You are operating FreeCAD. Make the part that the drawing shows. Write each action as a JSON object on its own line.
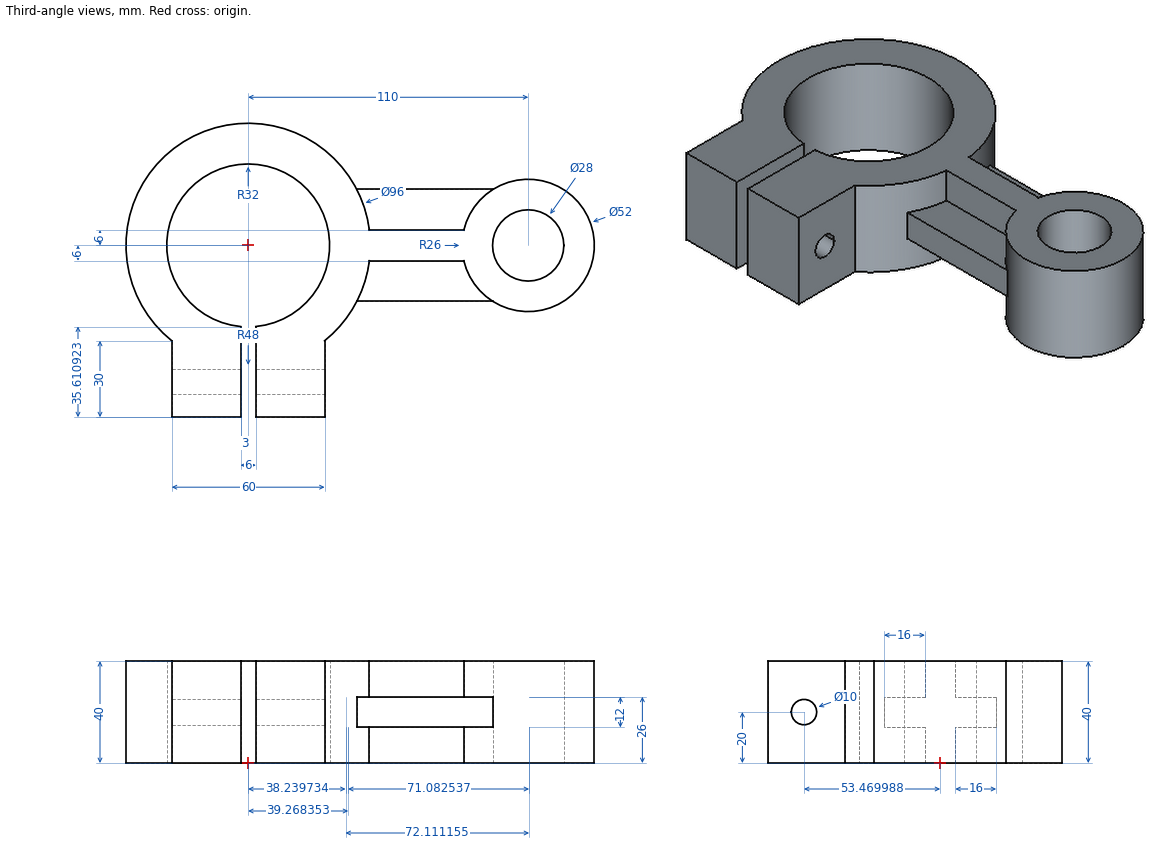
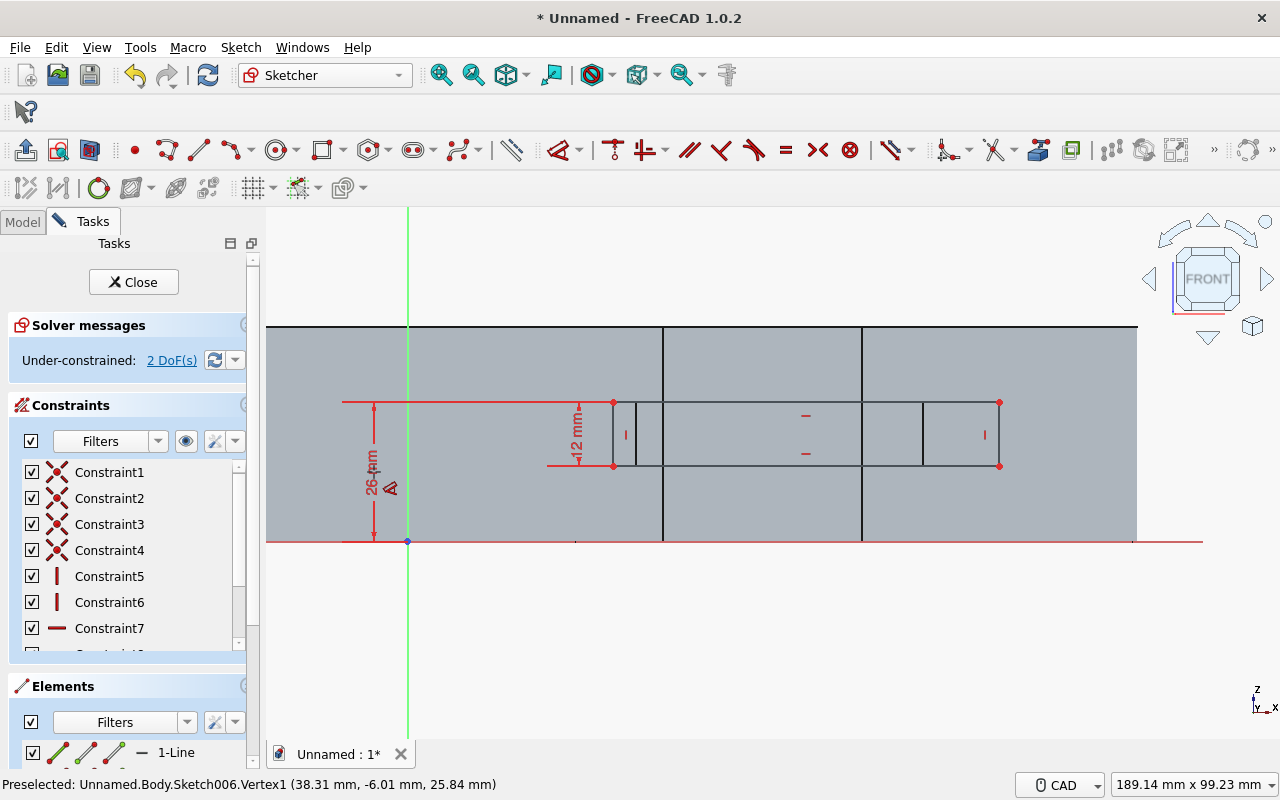
{"action": "left_click", "coordinate": [729, 466]}
{"action": "left_click", "coordinate": [806, 432]}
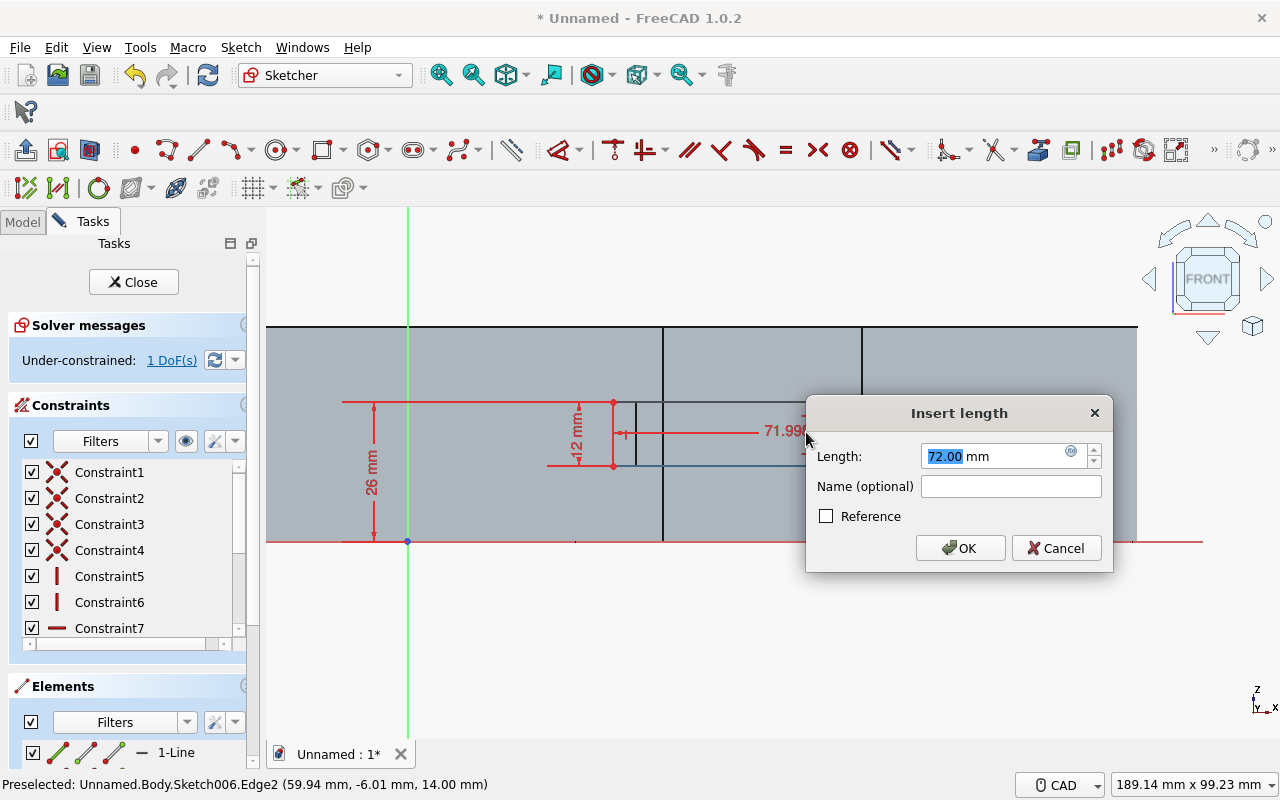
{"action": "type", "text": "72.111155"}
{"action": "key", "text": "Return"}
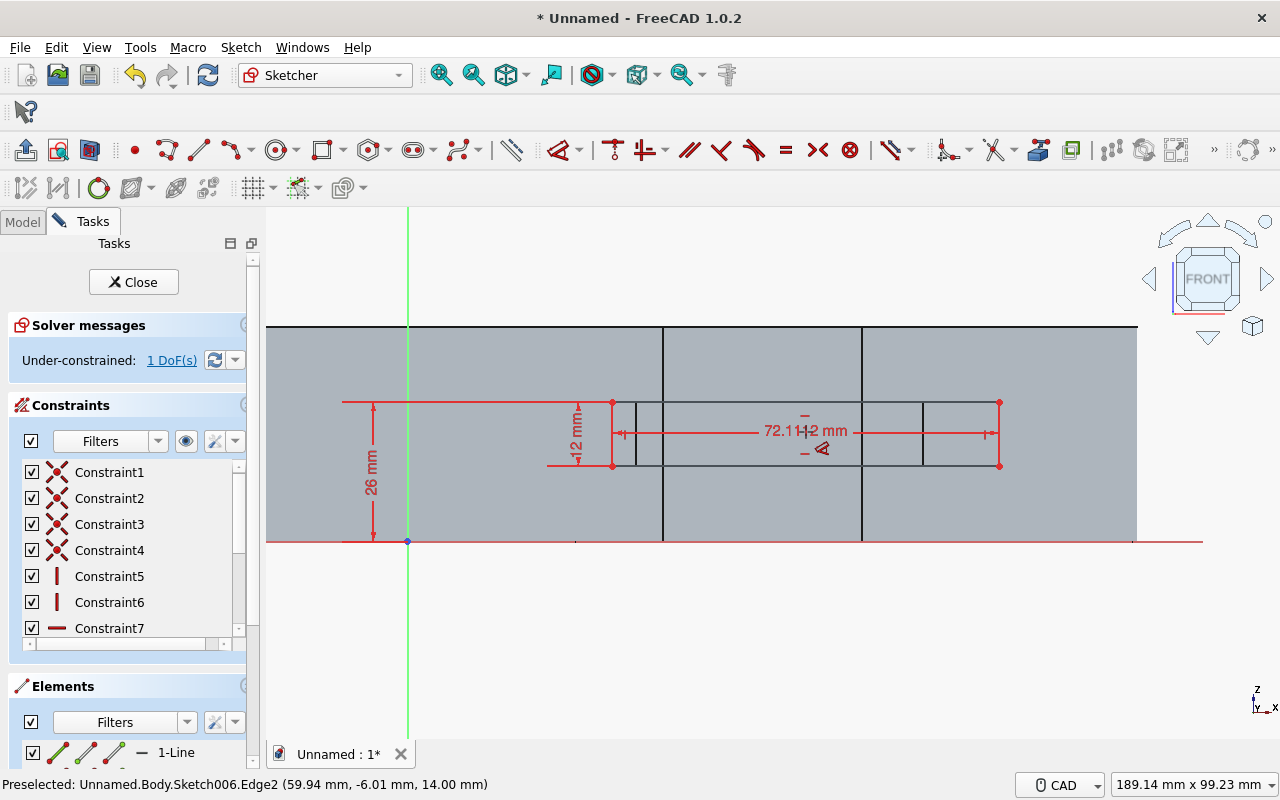
{"action": "left_click", "coordinate": [612, 402]}
{"action": "left_click", "coordinate": [510, 576]}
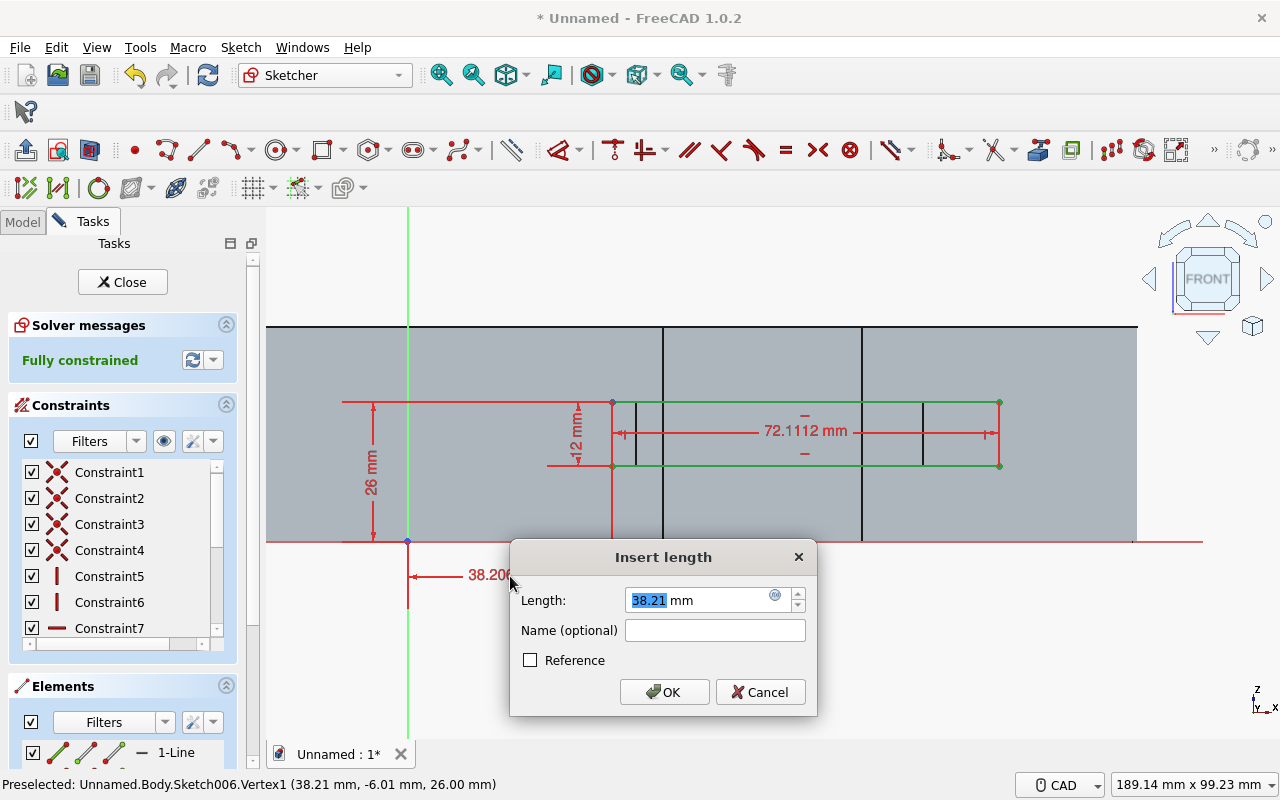
{"action": "type", "text": "38.239734"}
{"action": "key", "text": "Return"}
{"action": "key", "text": "Escape"}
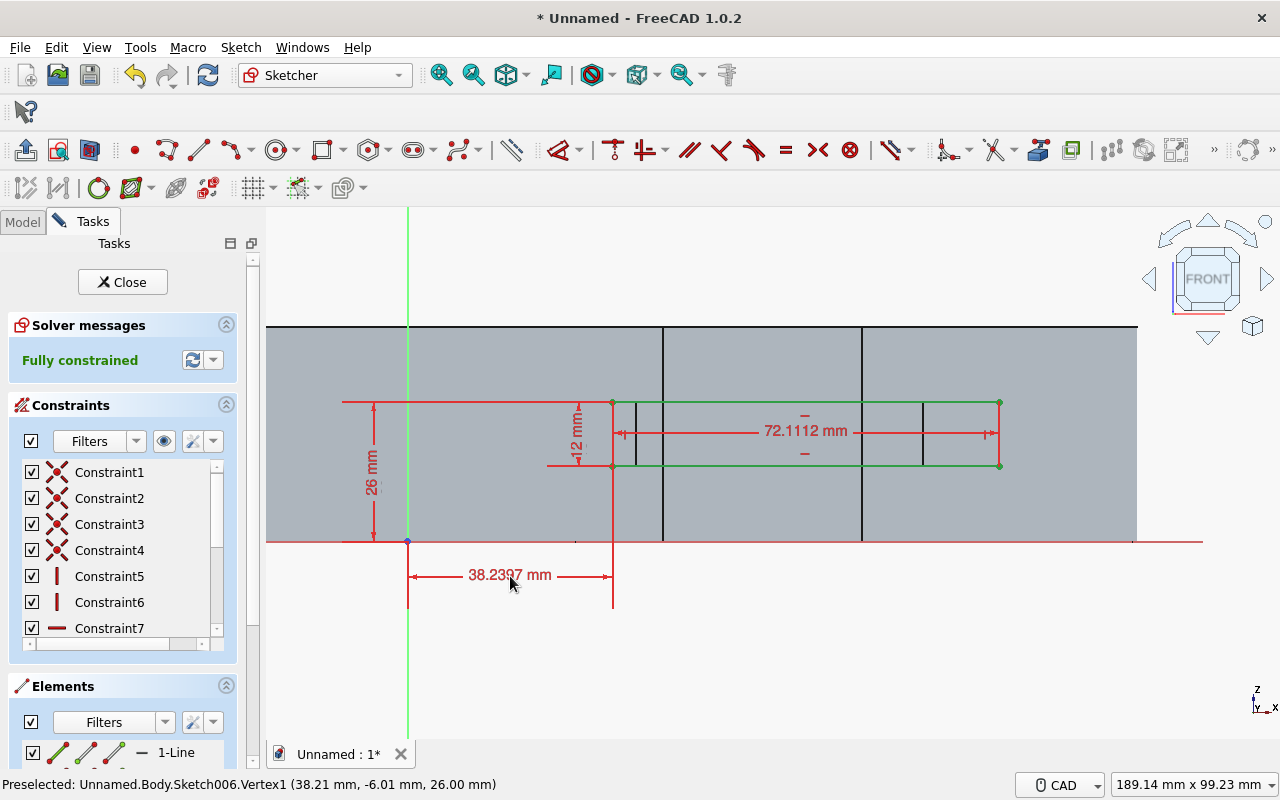
{"action": "left_click", "coordinate": [123, 282]}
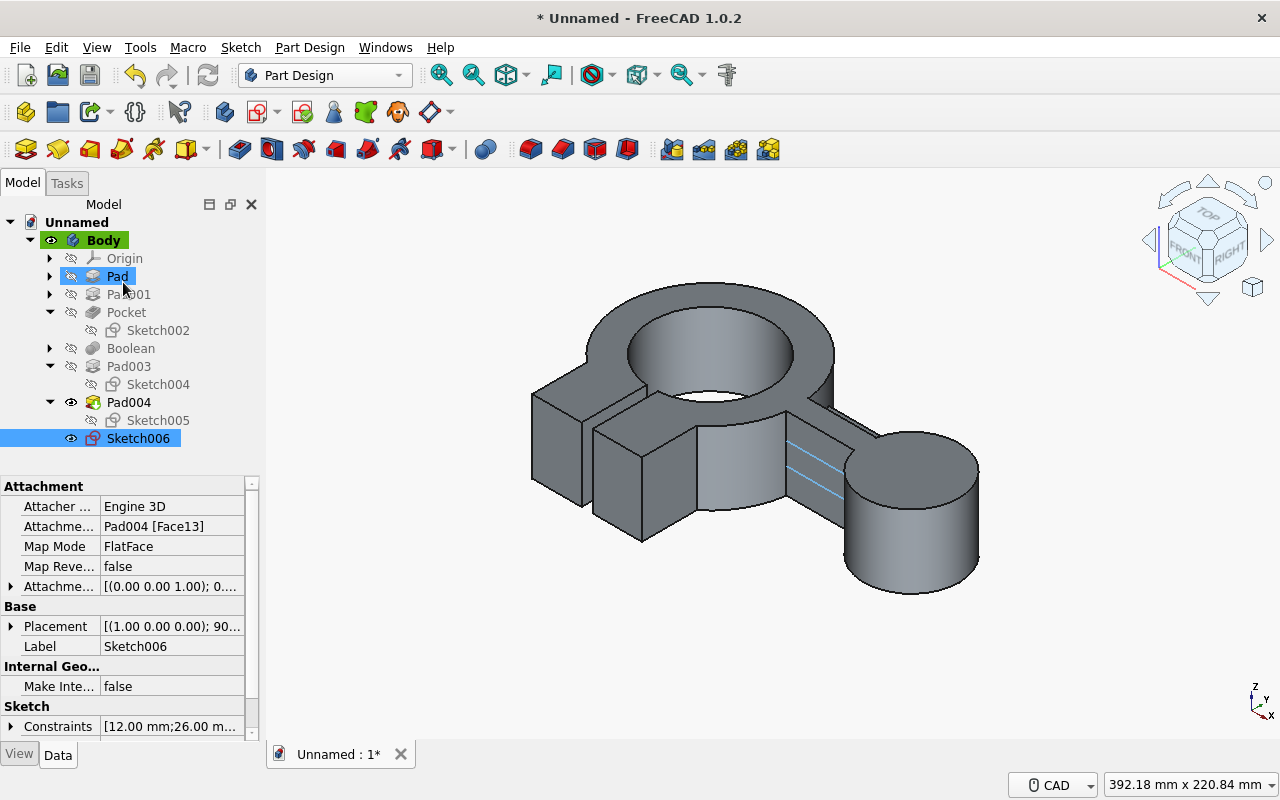
{"action": "left_click", "coordinate": [26, 150]}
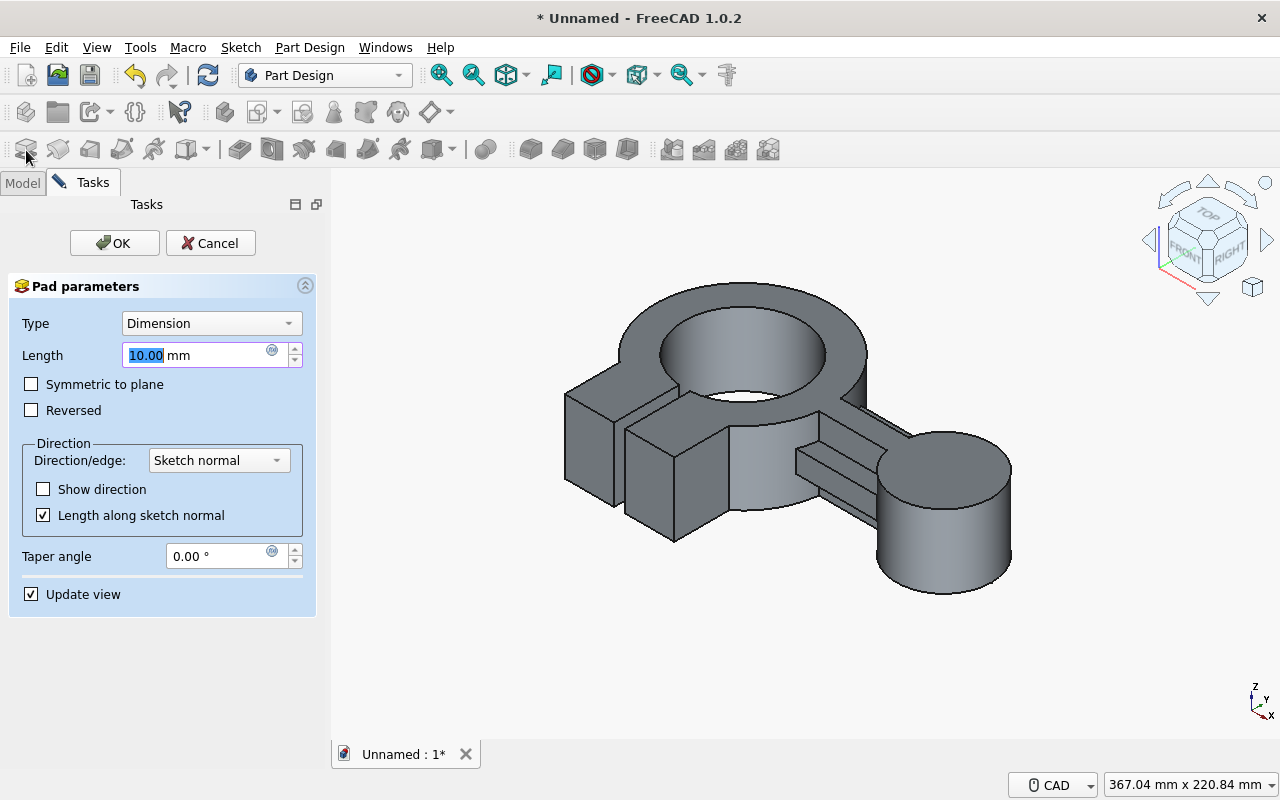
{"action": "type", "text": "16"}
{"action": "key", "text": "Tab"}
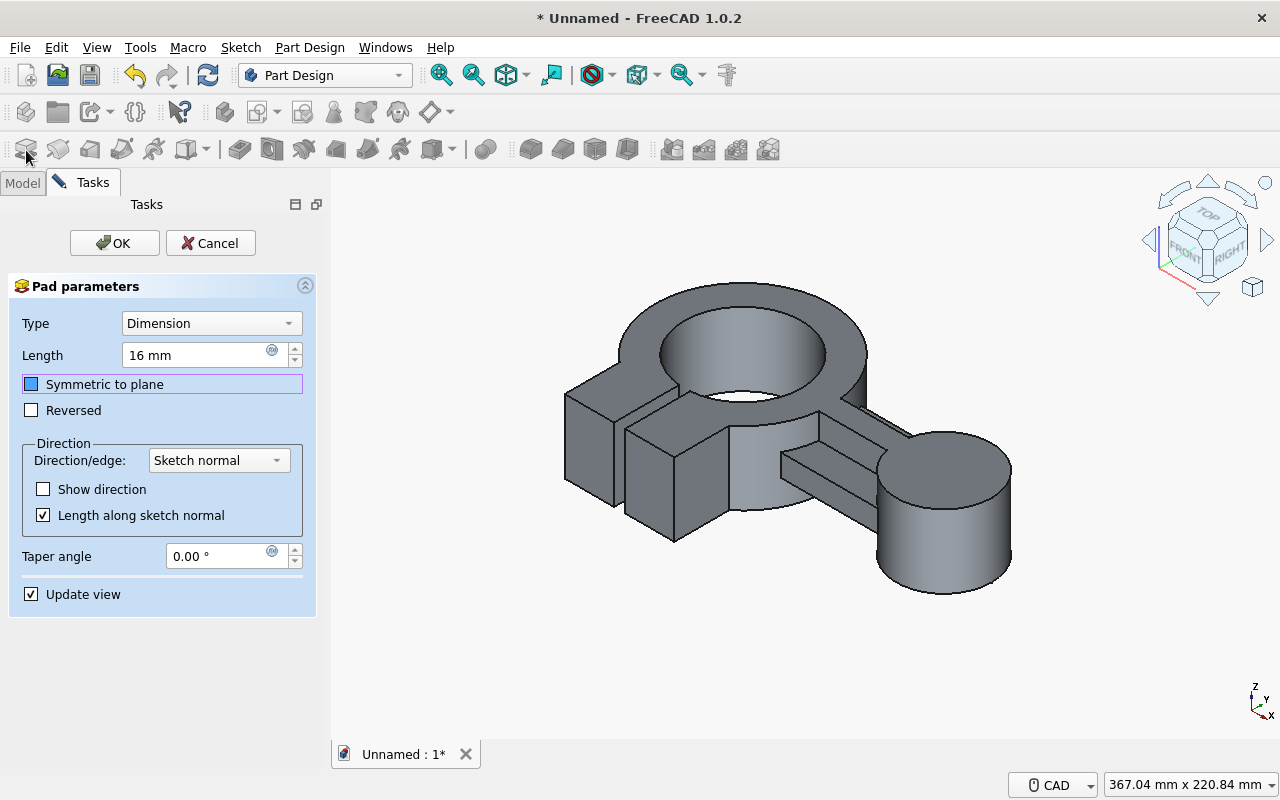
{"action": "left_click", "coordinate": [115, 243]}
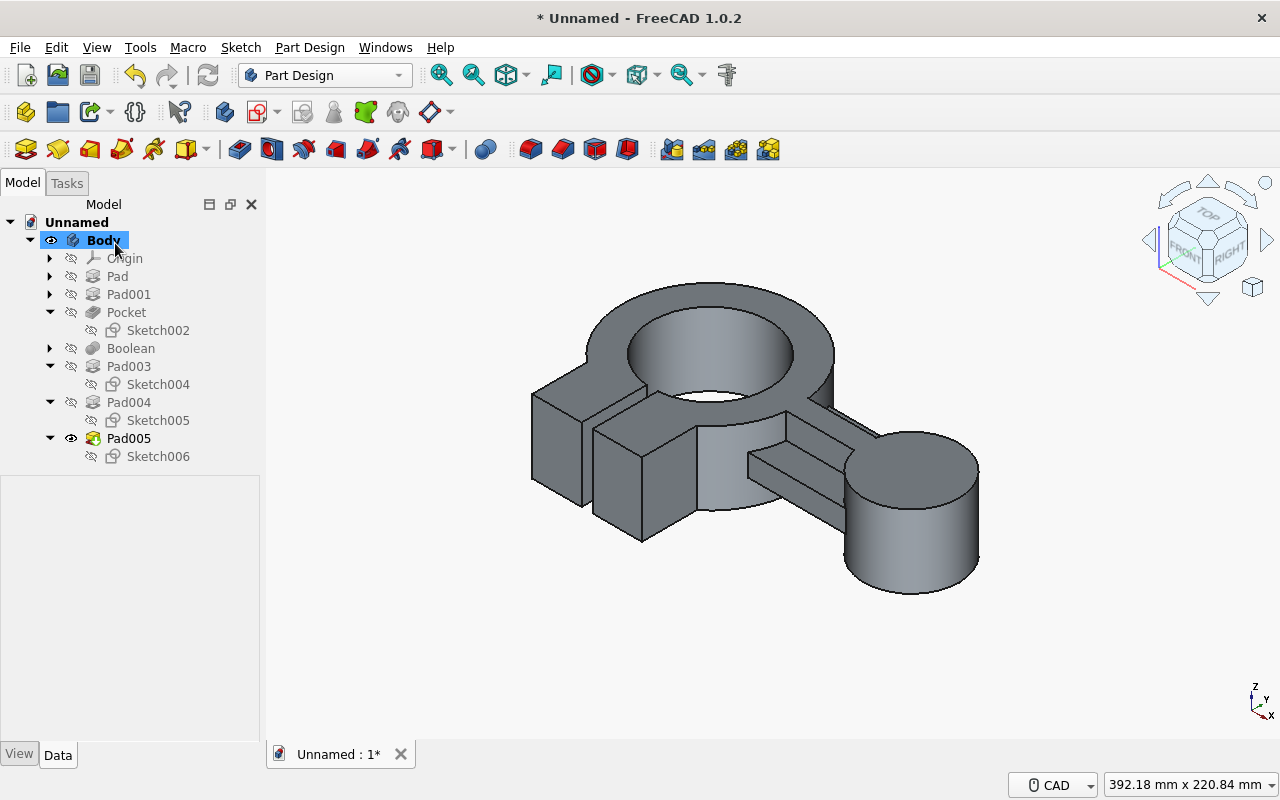
{"action": "left_click", "coordinate": [665, 417]}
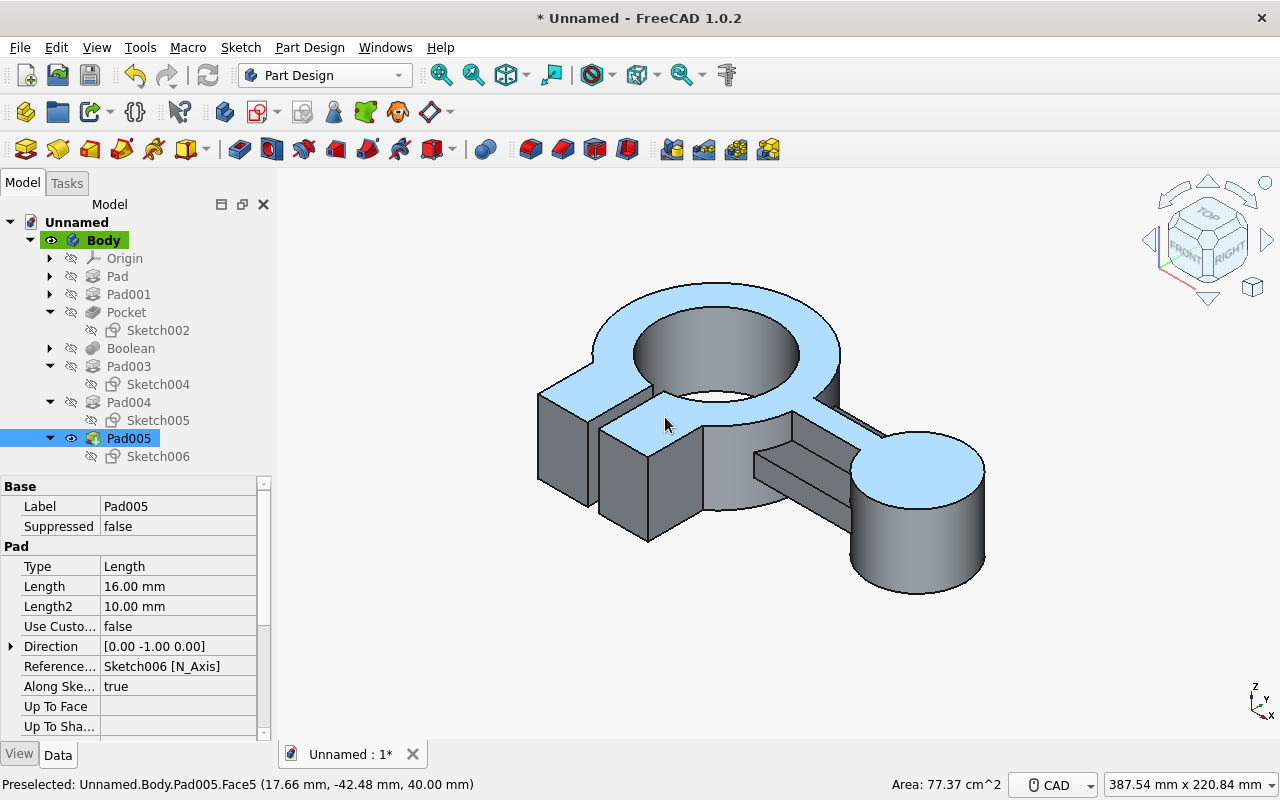
{"action": "left_click", "coordinate": [258, 112]}